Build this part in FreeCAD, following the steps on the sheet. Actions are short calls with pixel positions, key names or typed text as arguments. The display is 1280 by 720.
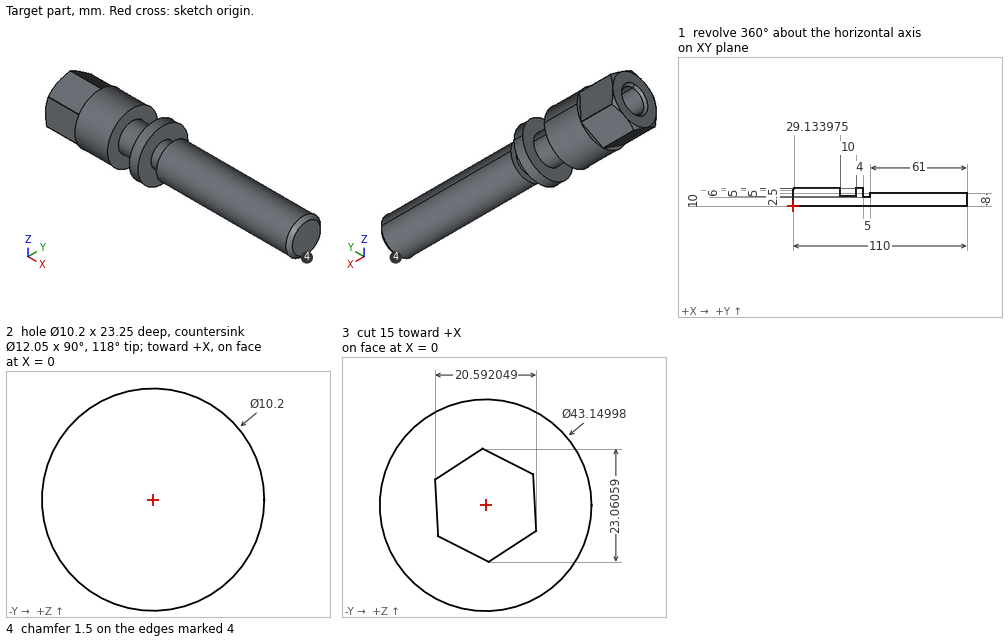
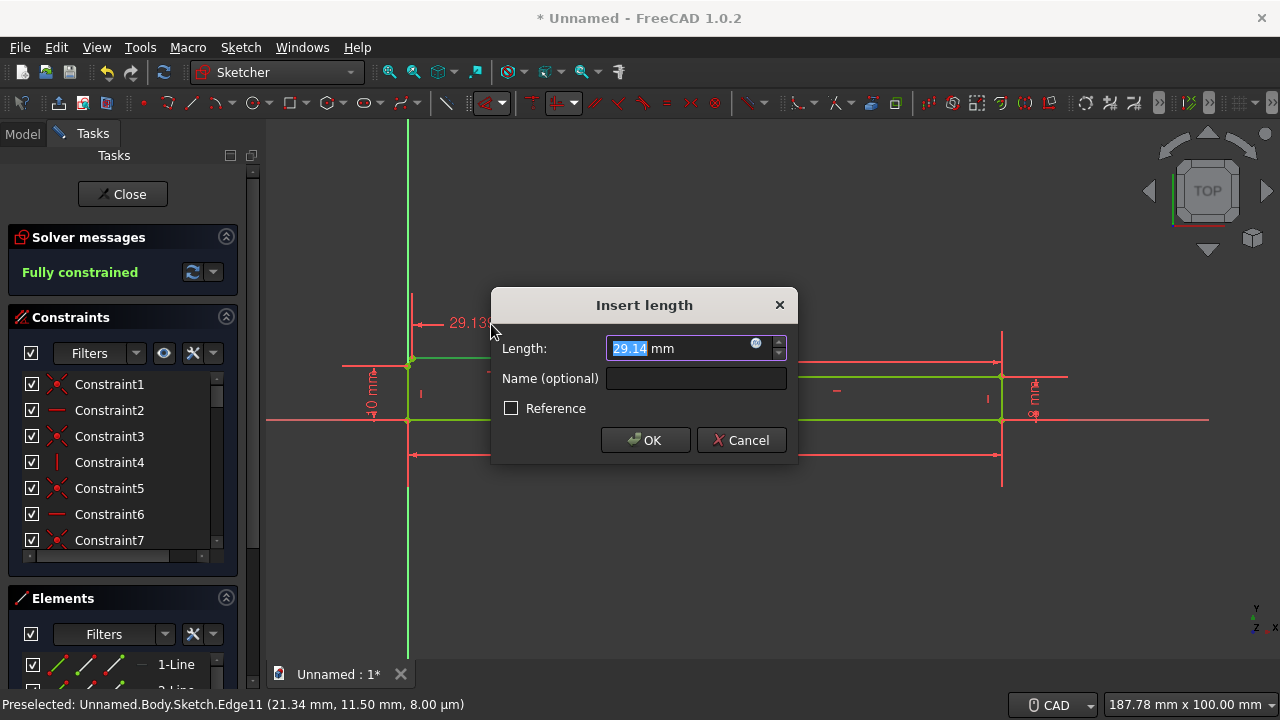
text(29.133975)
key(Return)
key(Escape)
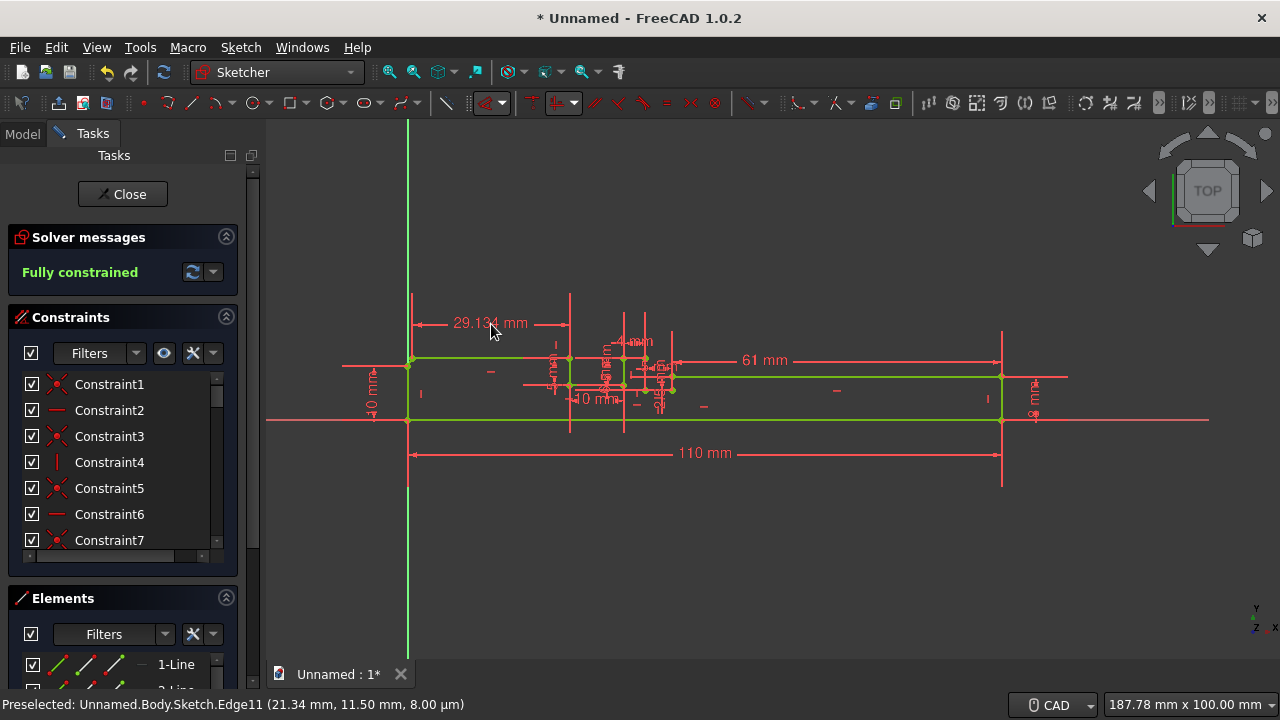
click(123, 194)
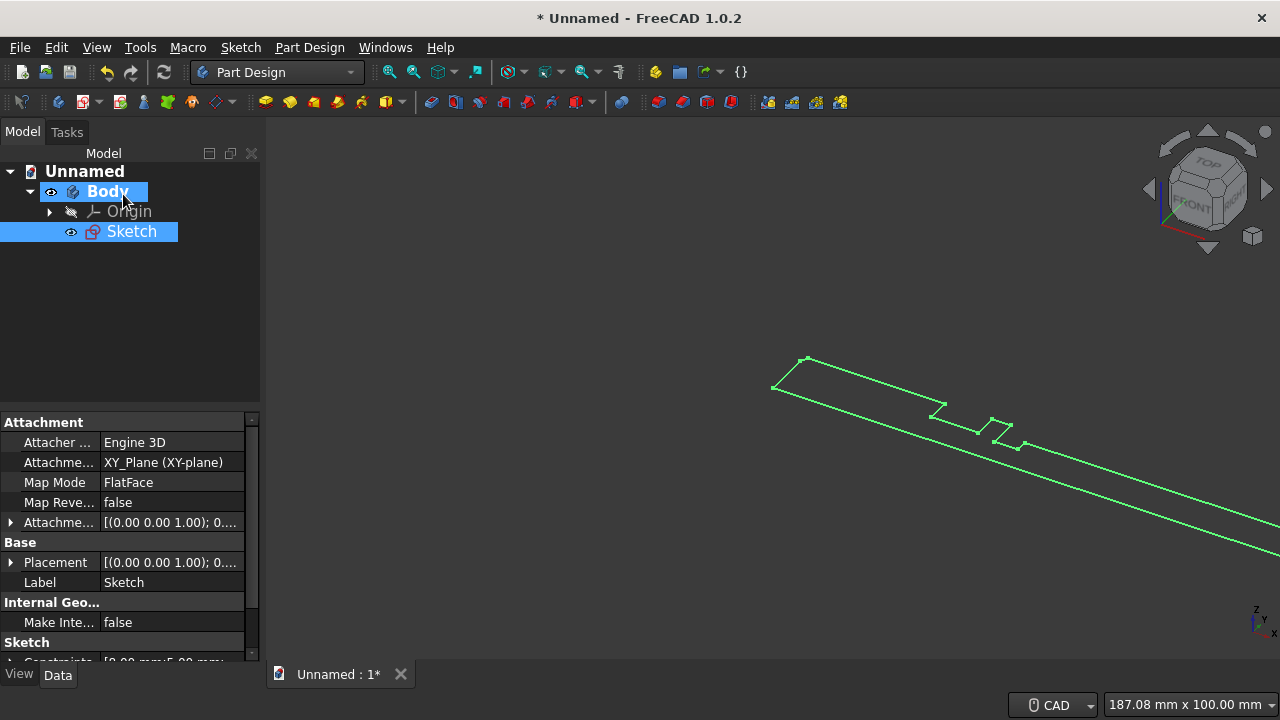
click(290, 102)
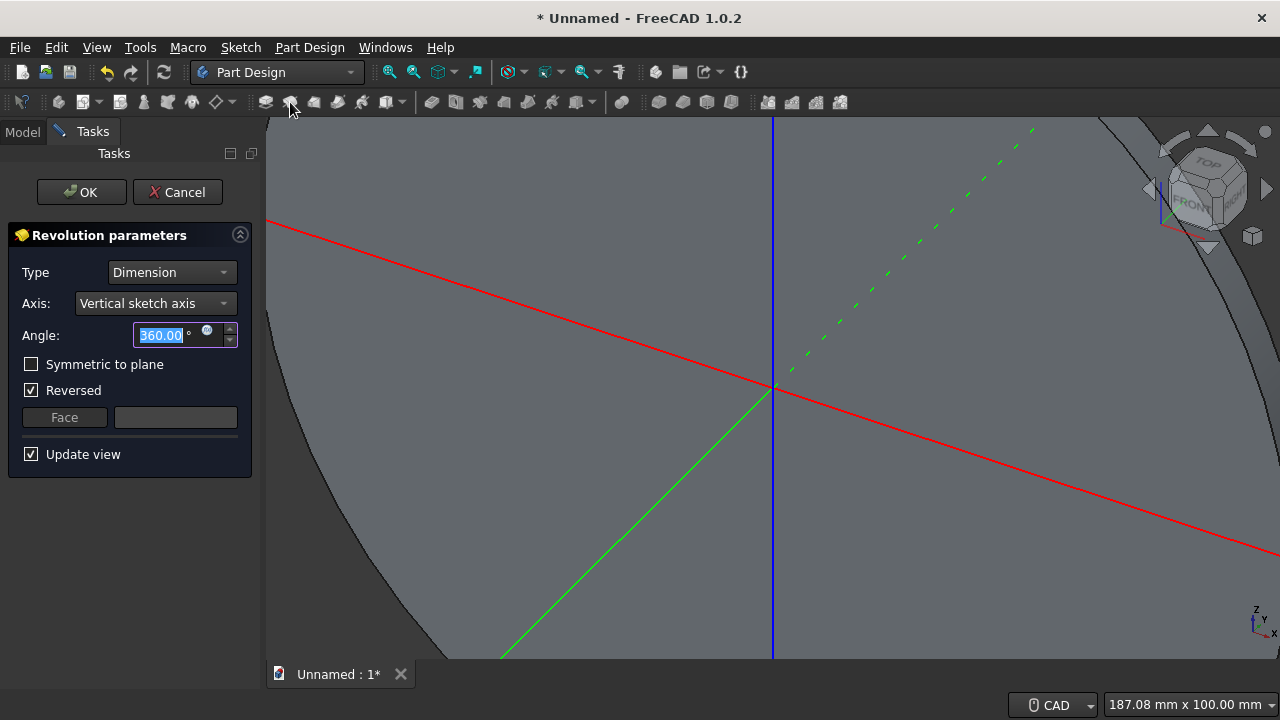
click(156, 304)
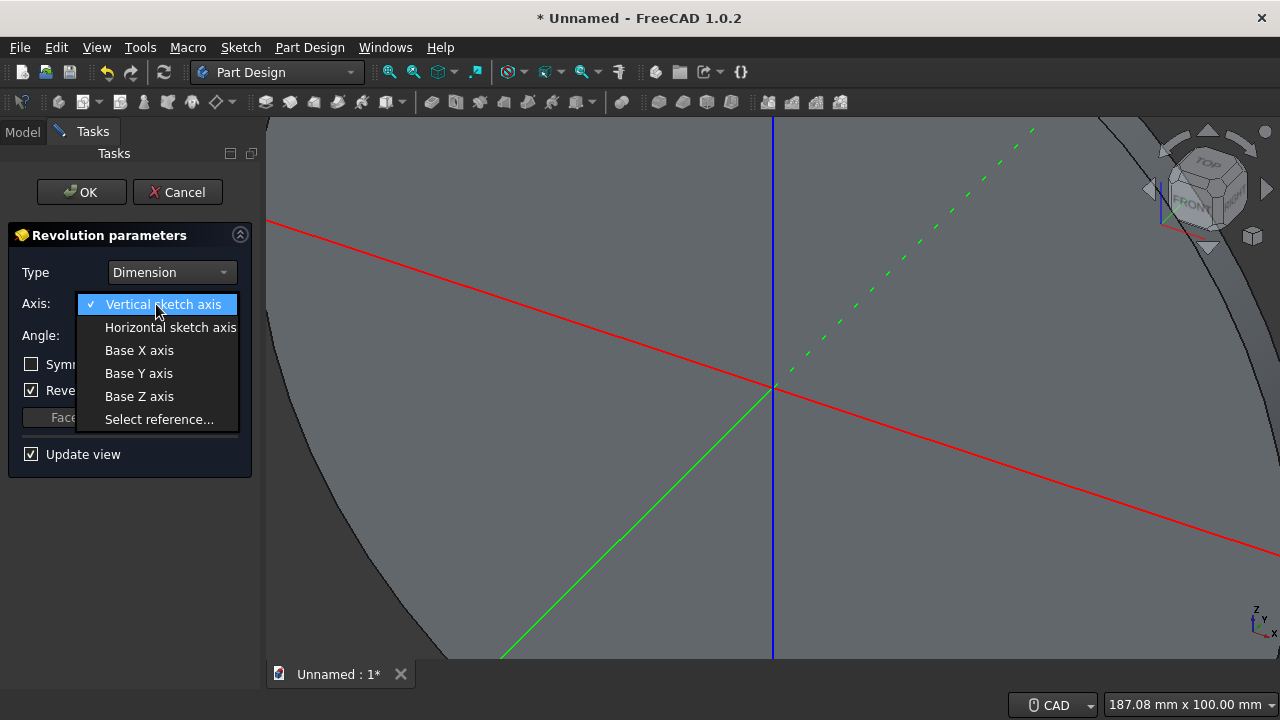
click(156, 328)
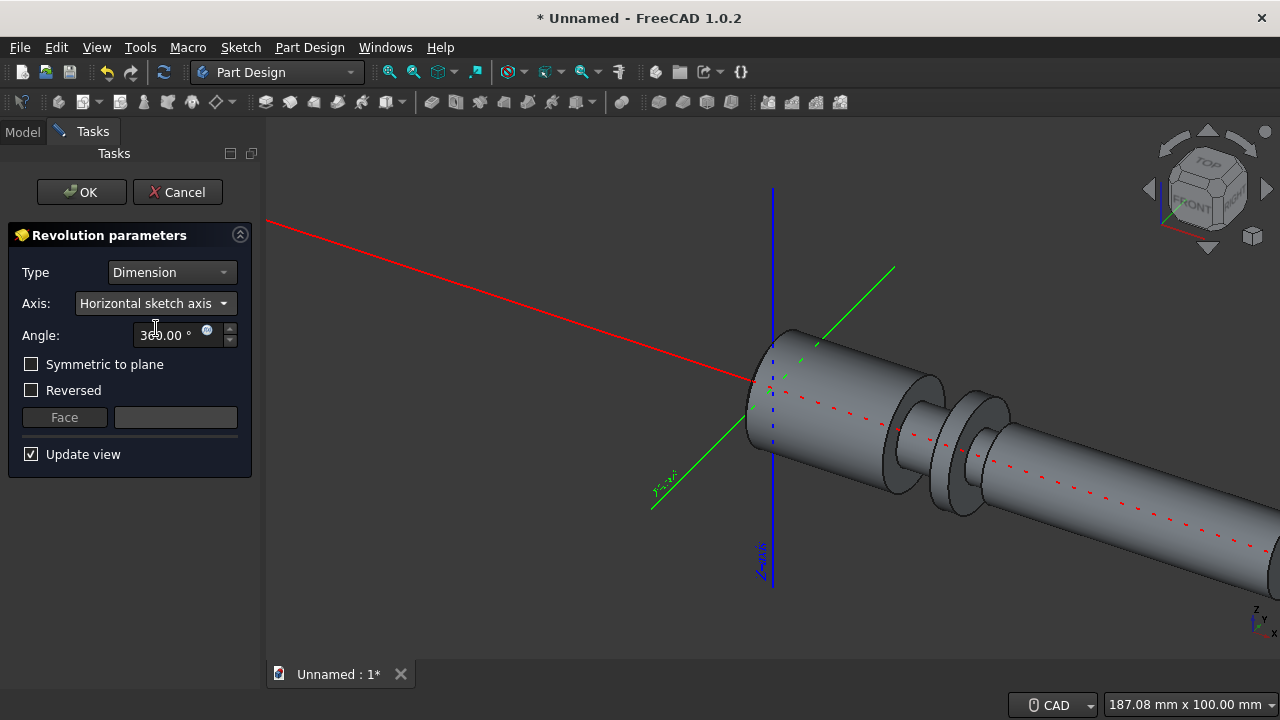
click(82, 192)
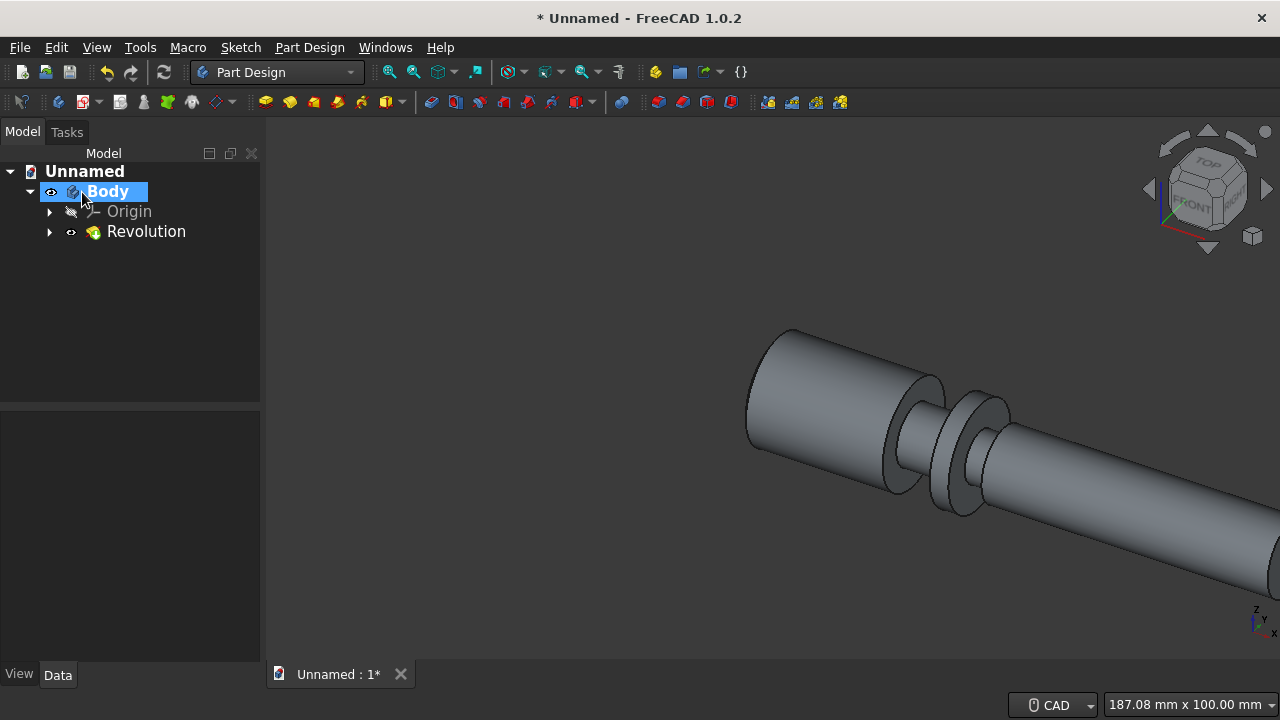
key(v)
key(f)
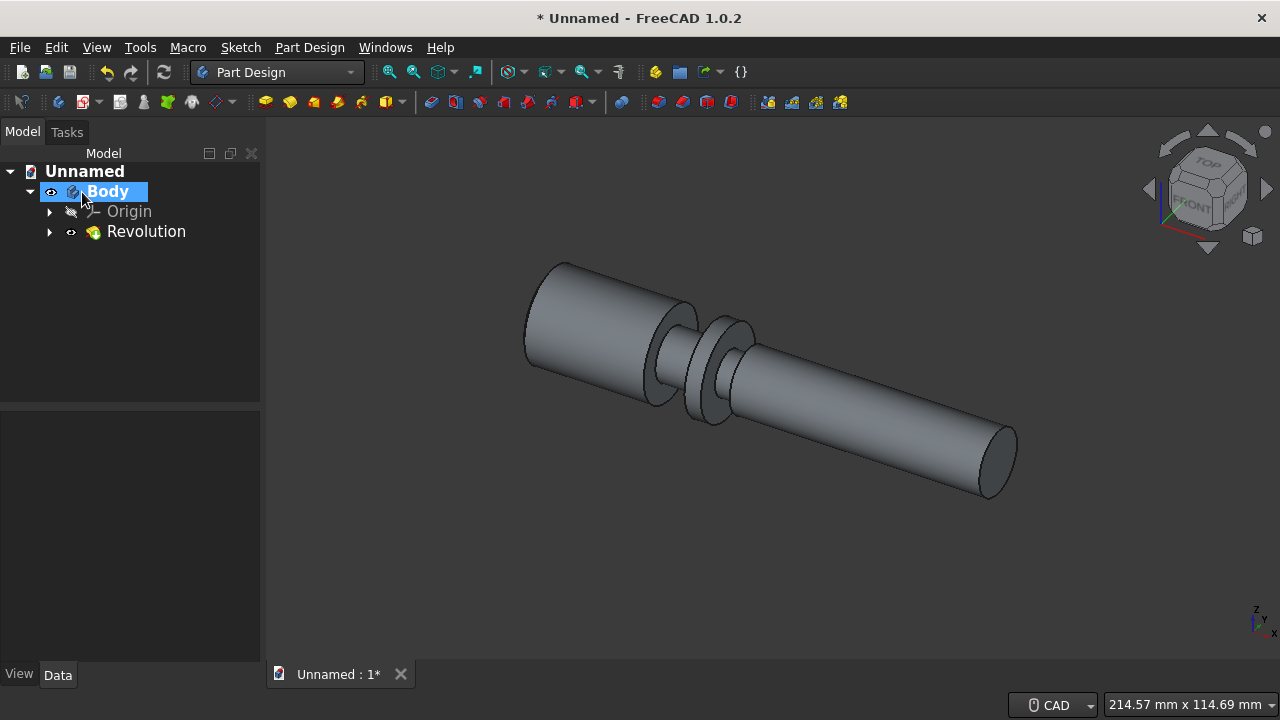
key(6)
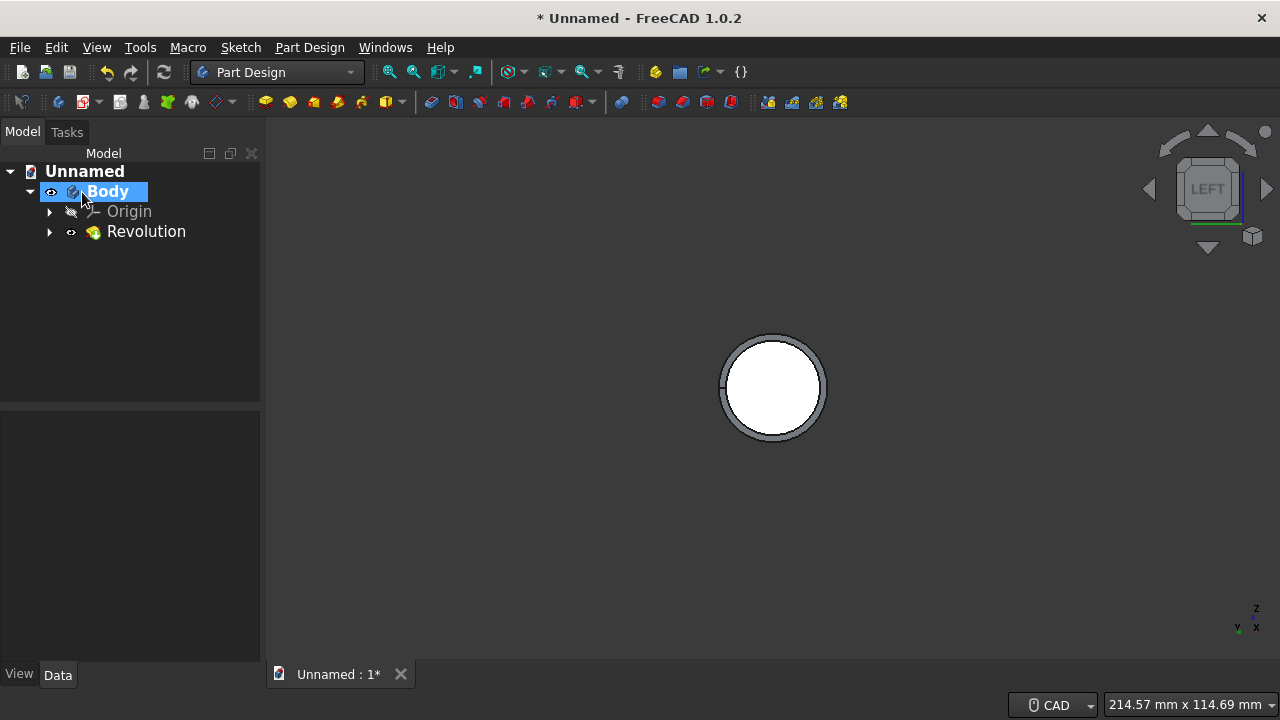
click(390, 72)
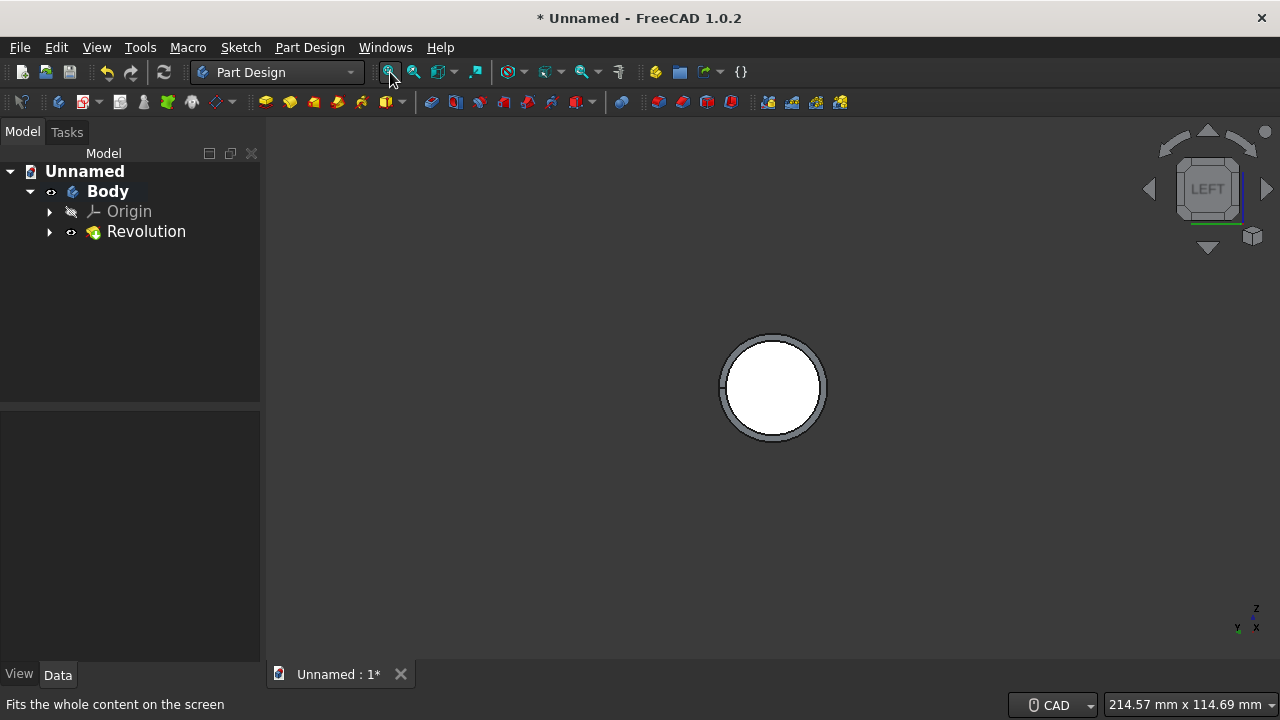
click(773, 387)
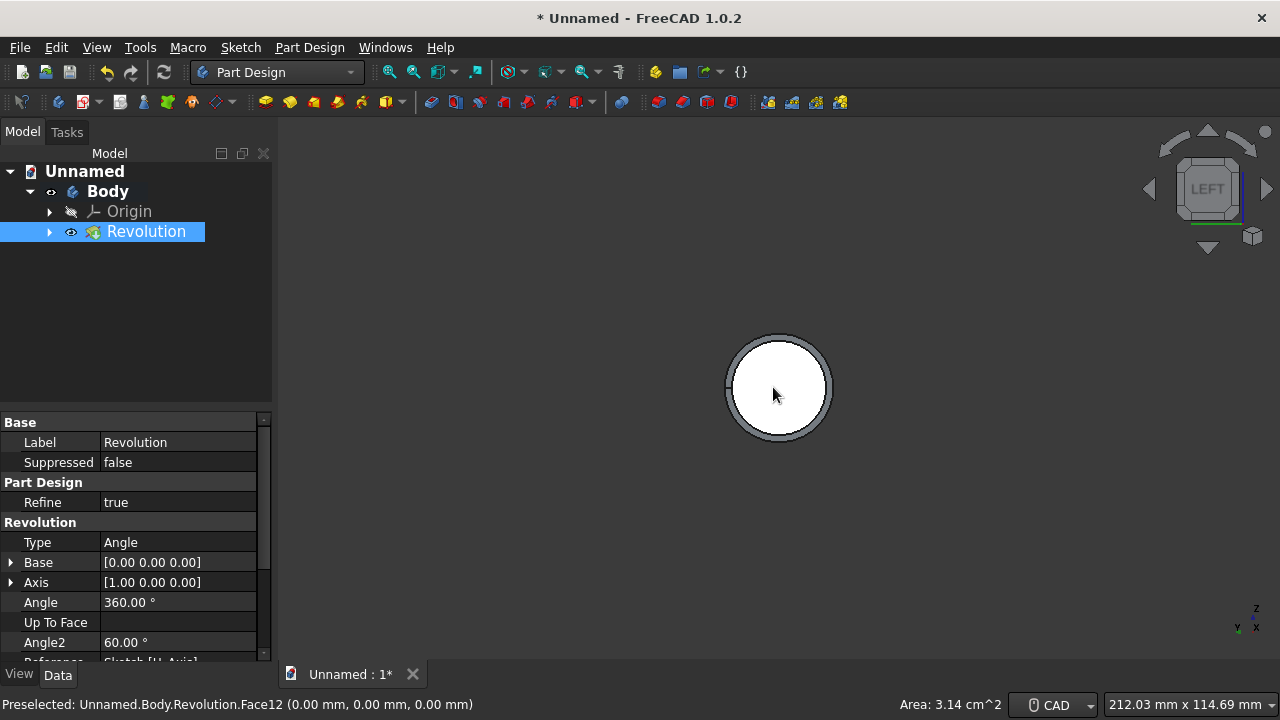
click(84, 102)